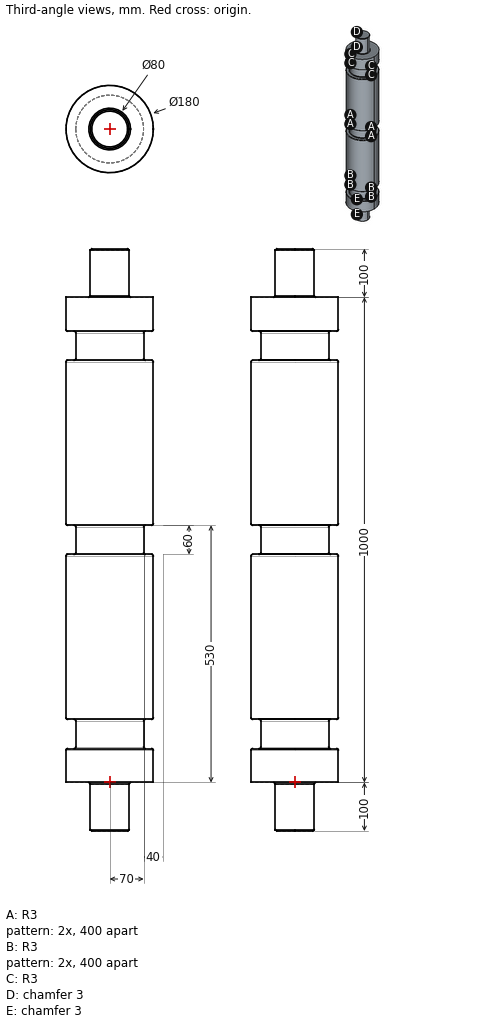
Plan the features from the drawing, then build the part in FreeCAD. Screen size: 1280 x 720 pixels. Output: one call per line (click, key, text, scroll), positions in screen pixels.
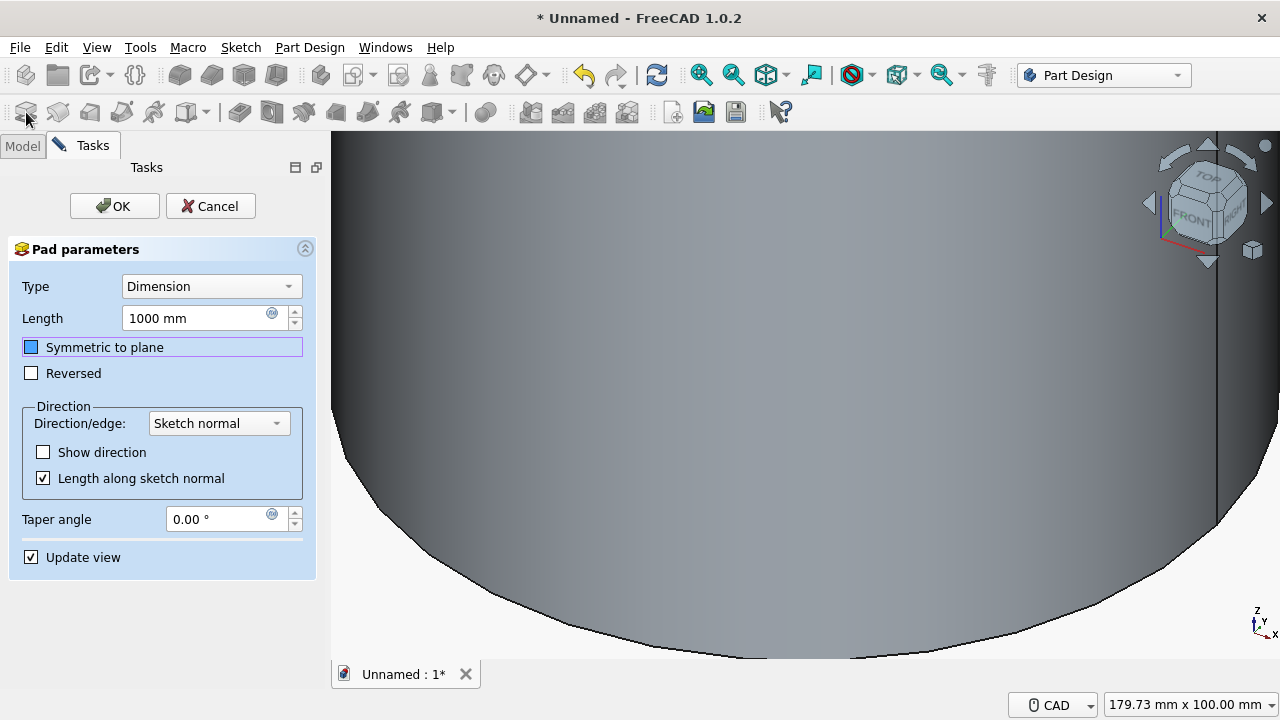
click(115, 206)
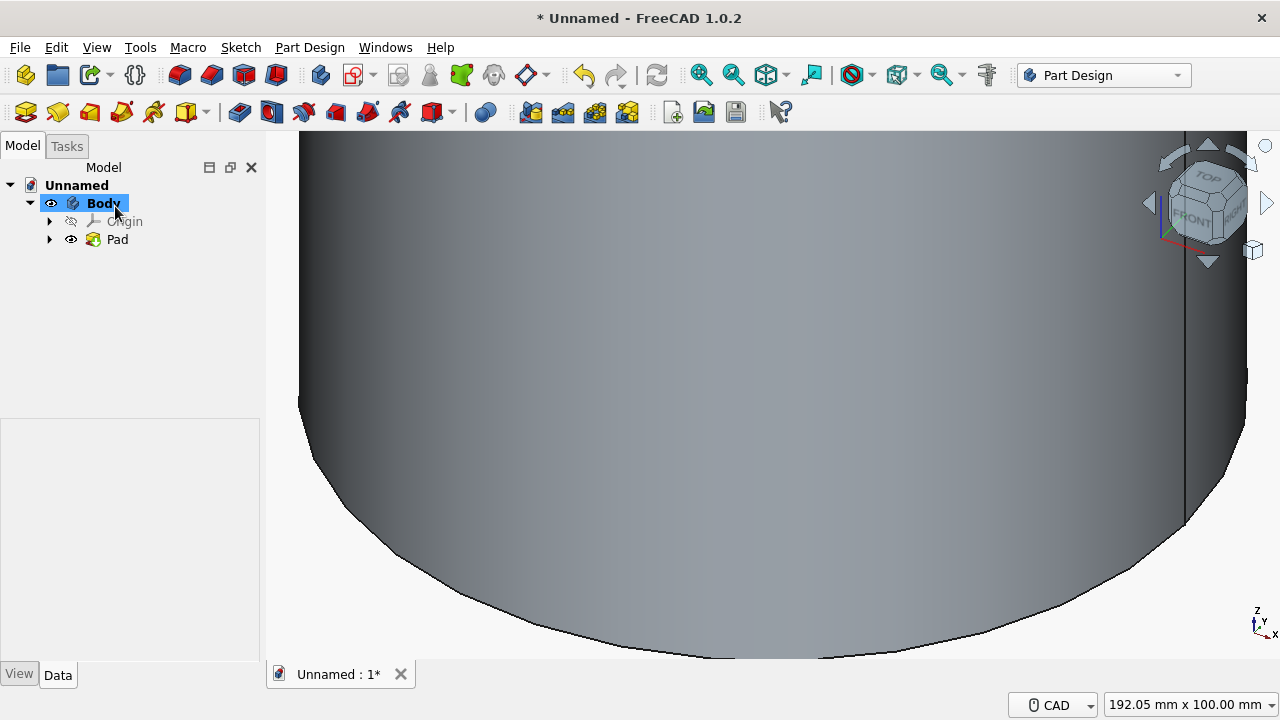
click(702, 76)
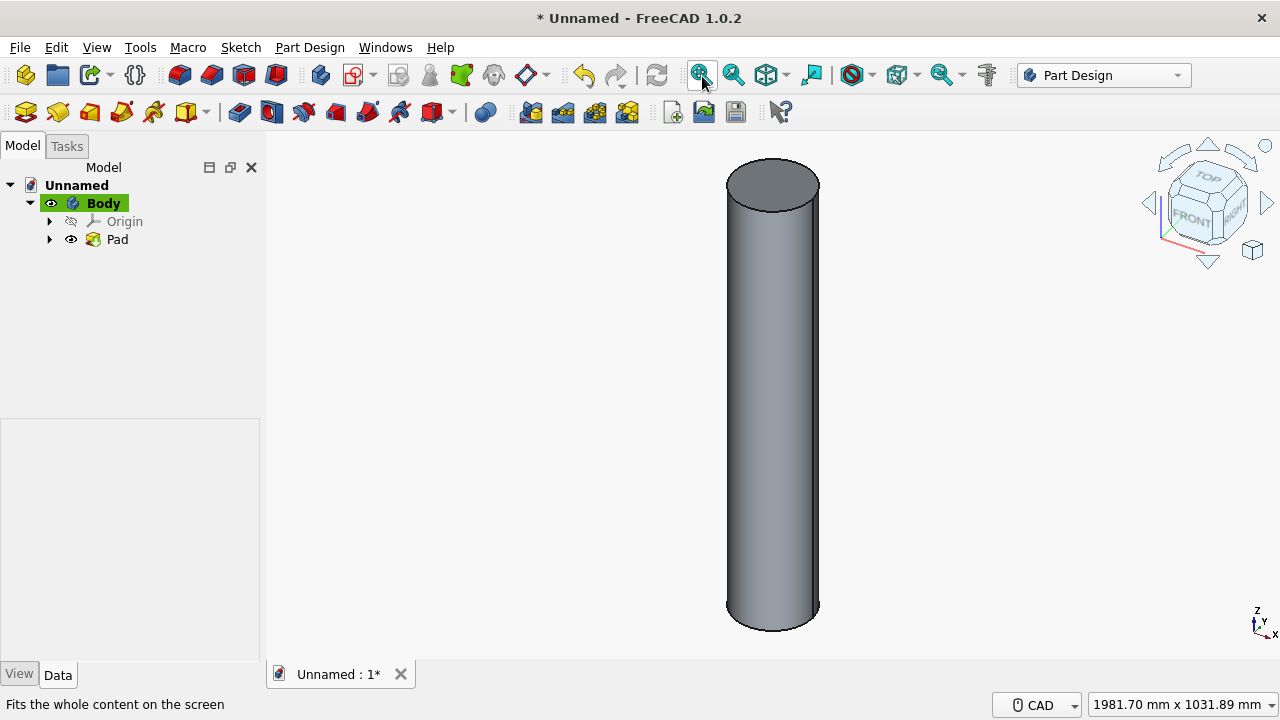
click(354, 76)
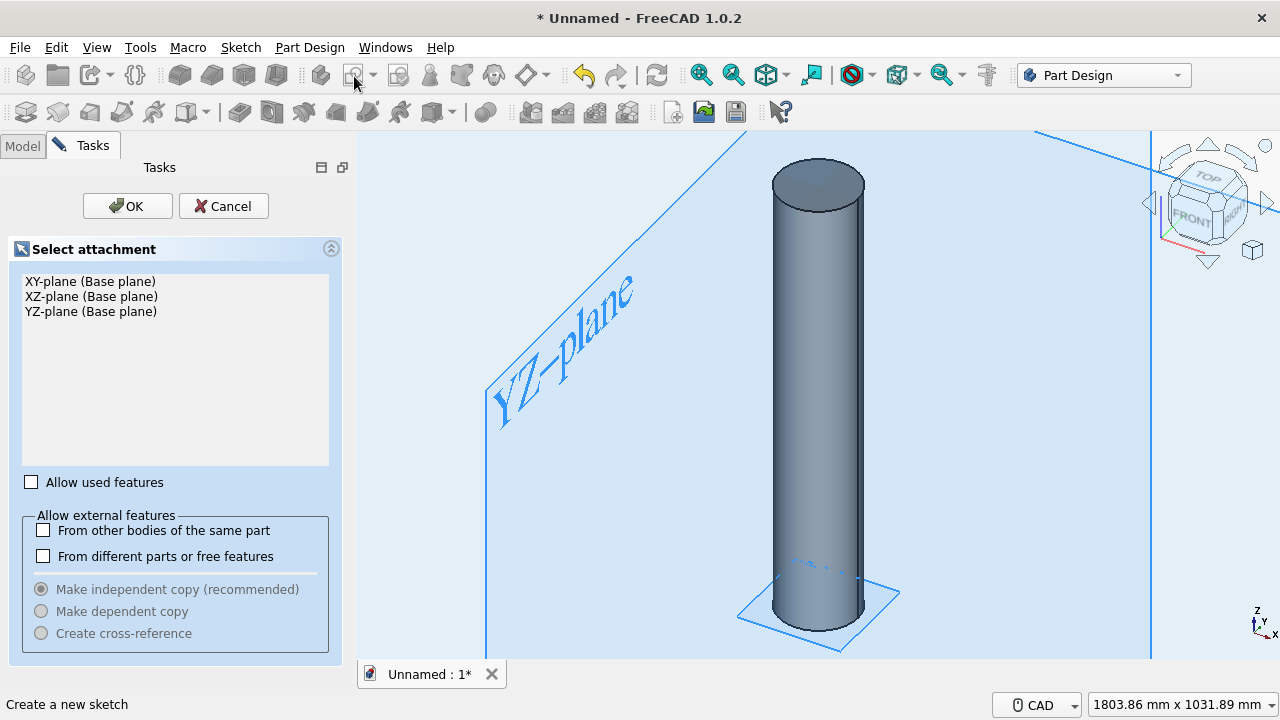
click(82, 296)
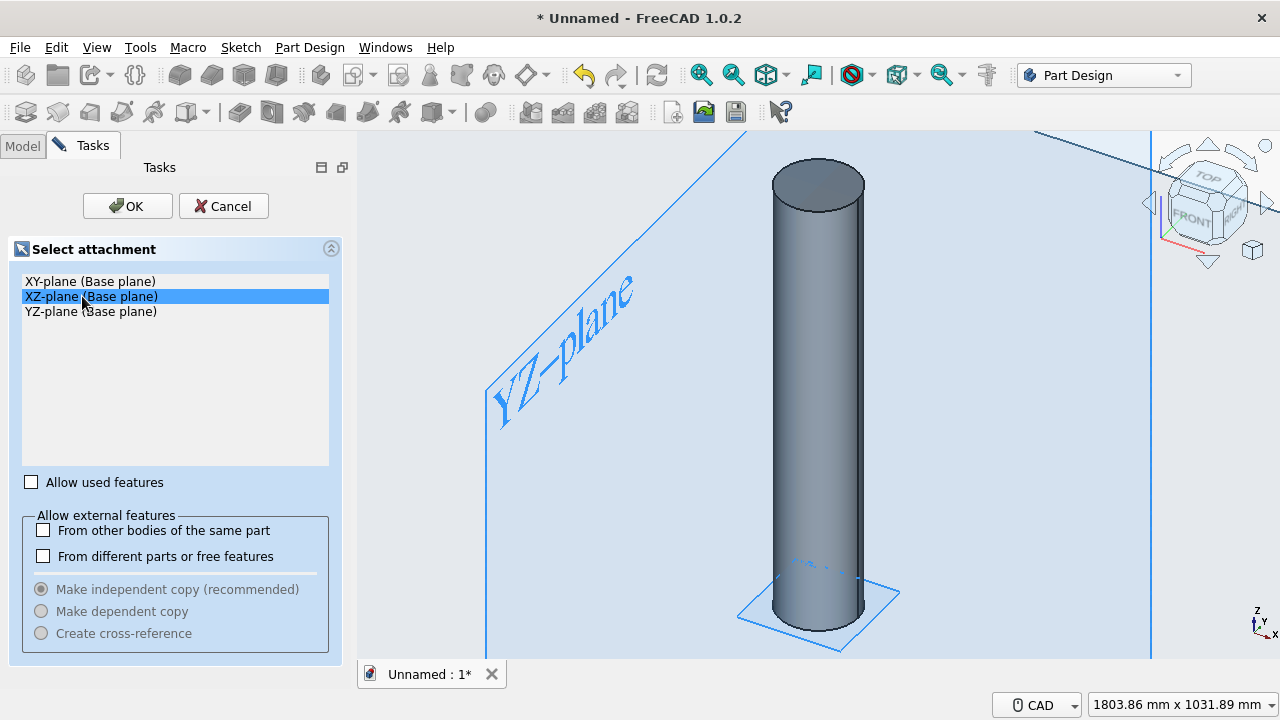
click(128, 206)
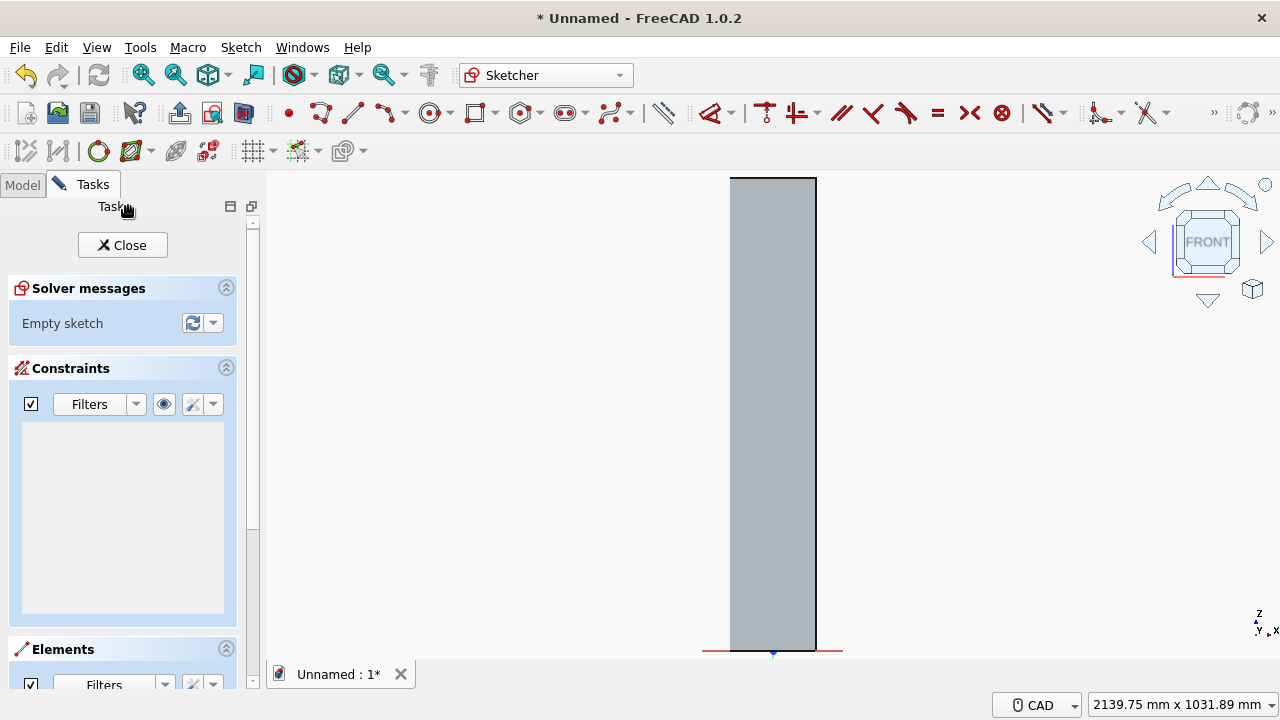
click(244, 114)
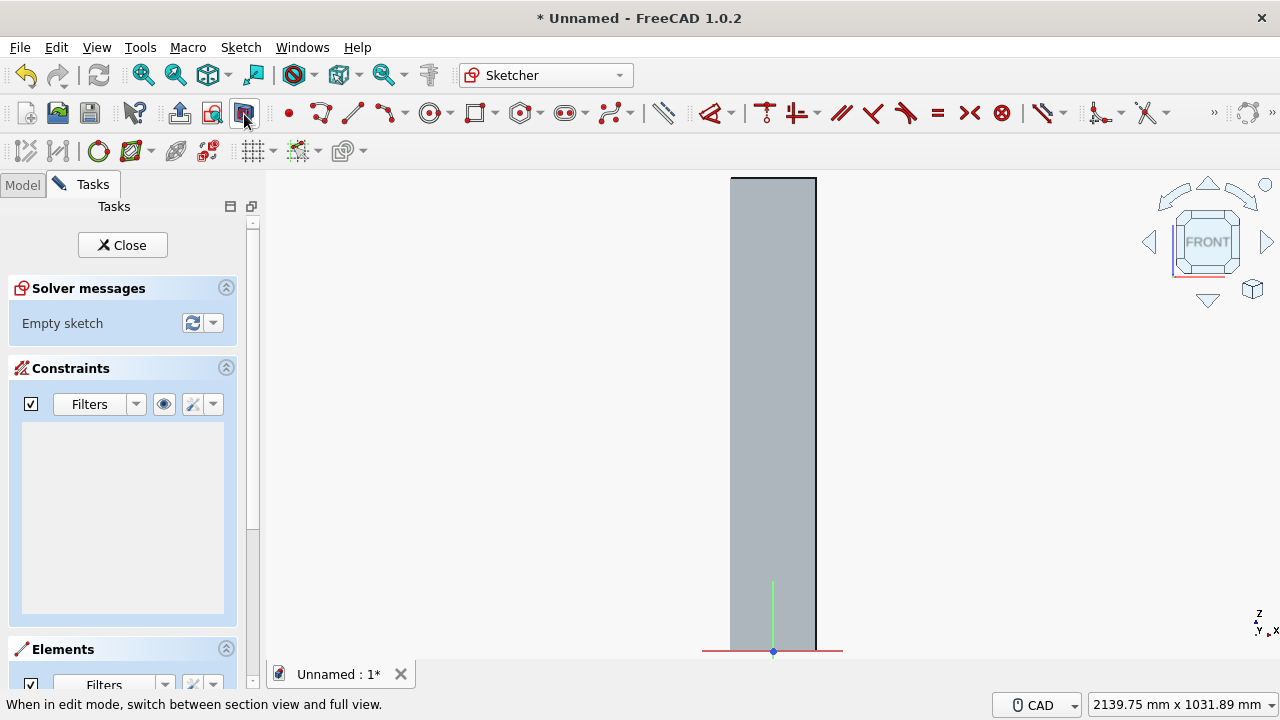
scroll(827, 414, up, 12)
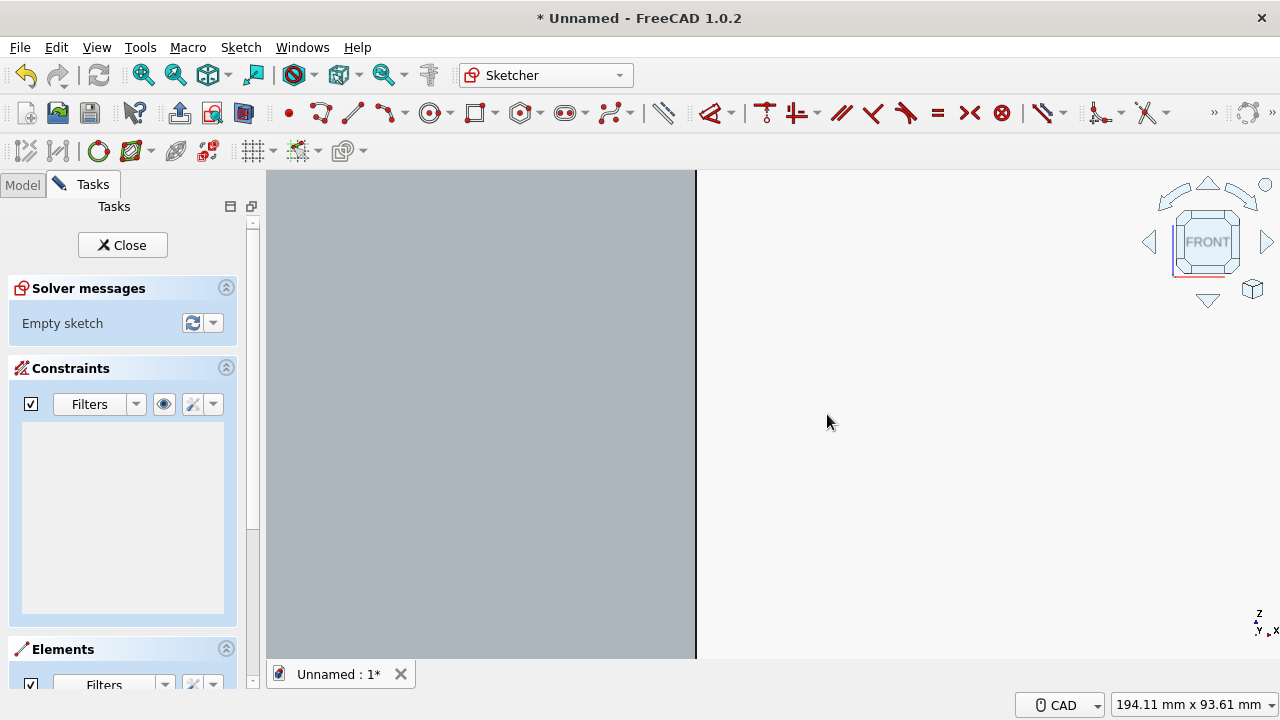
click(476, 114)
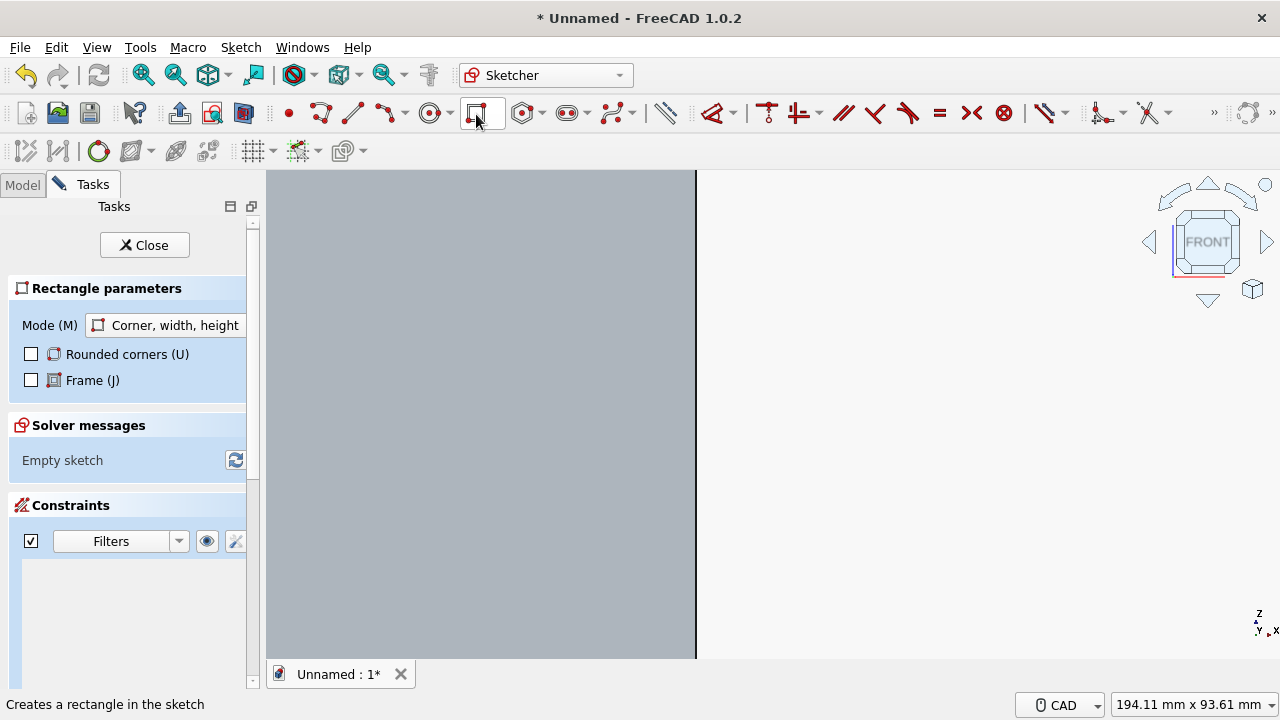
click(592, 258)
move(801, 571)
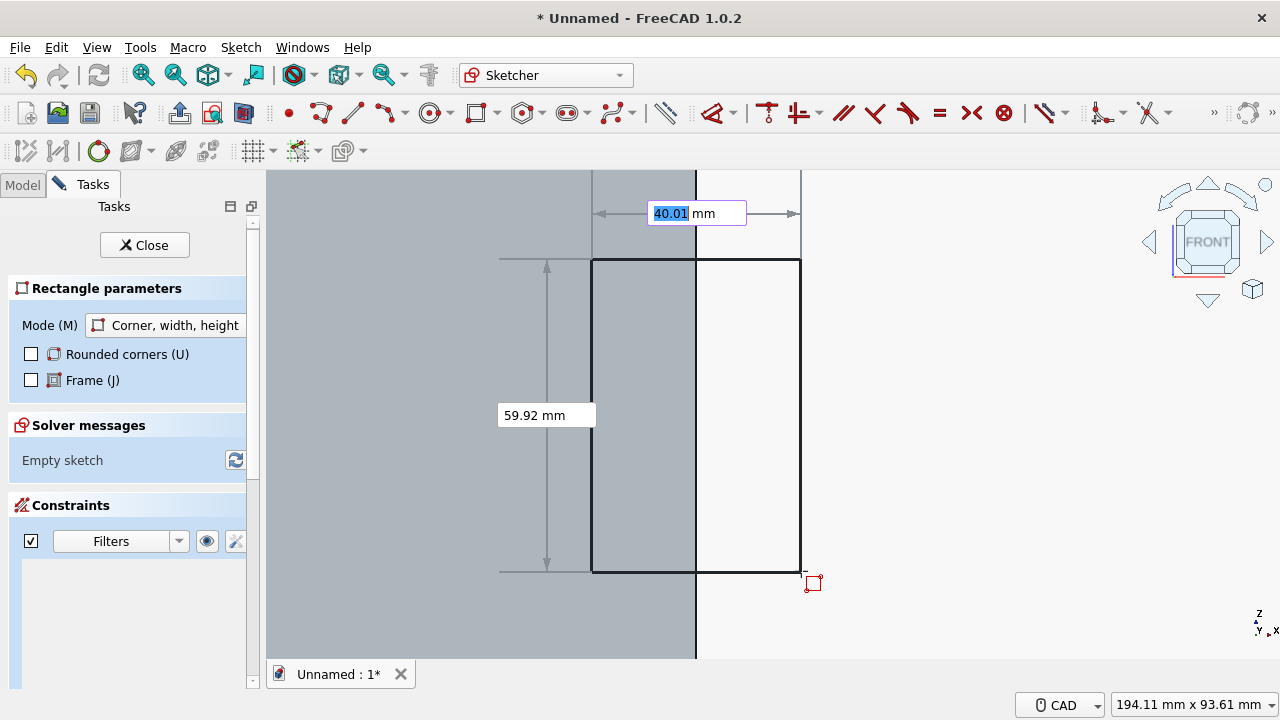
text(40)
key(Tab)
text(60)
key(Return)
key(Escape)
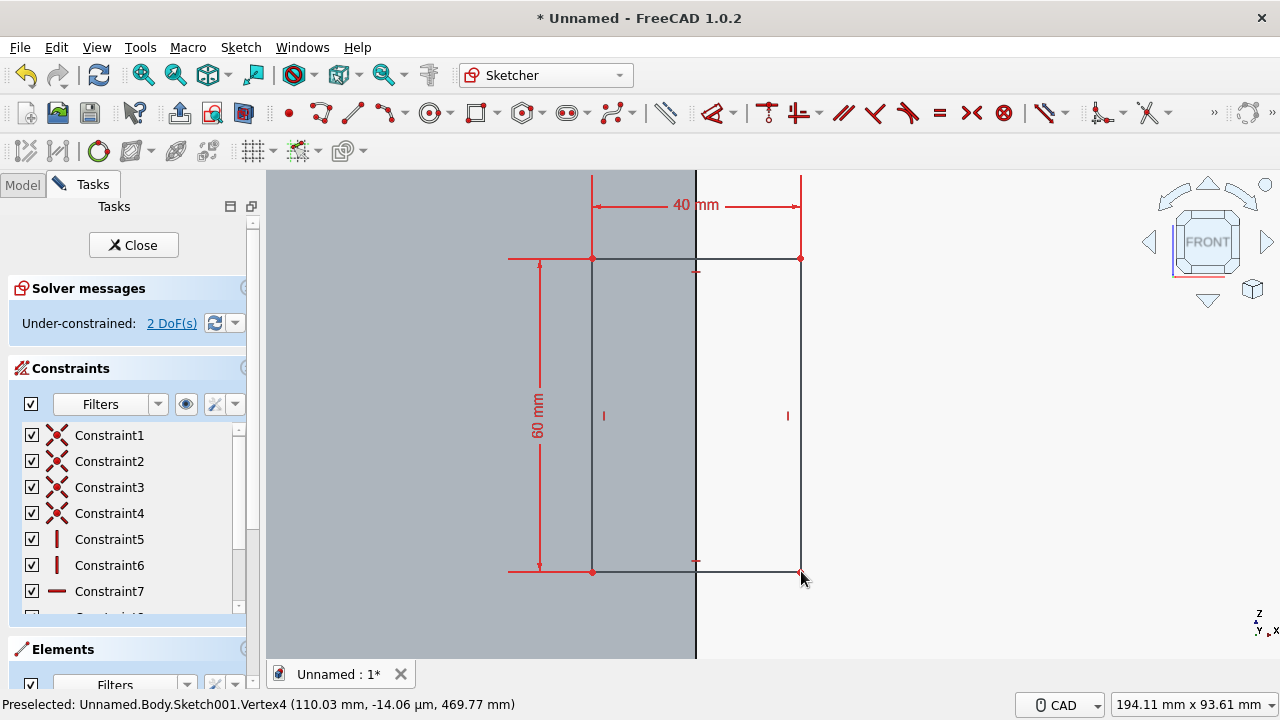
click(712, 114)